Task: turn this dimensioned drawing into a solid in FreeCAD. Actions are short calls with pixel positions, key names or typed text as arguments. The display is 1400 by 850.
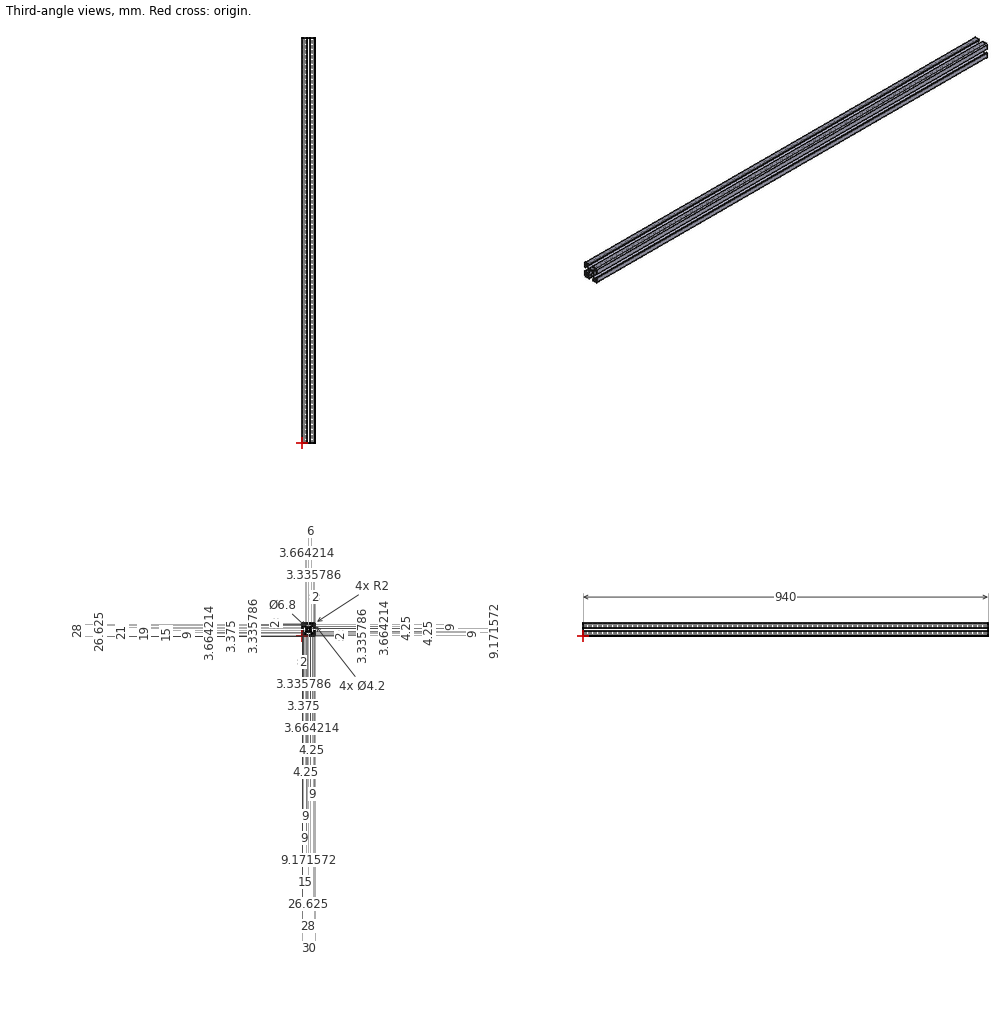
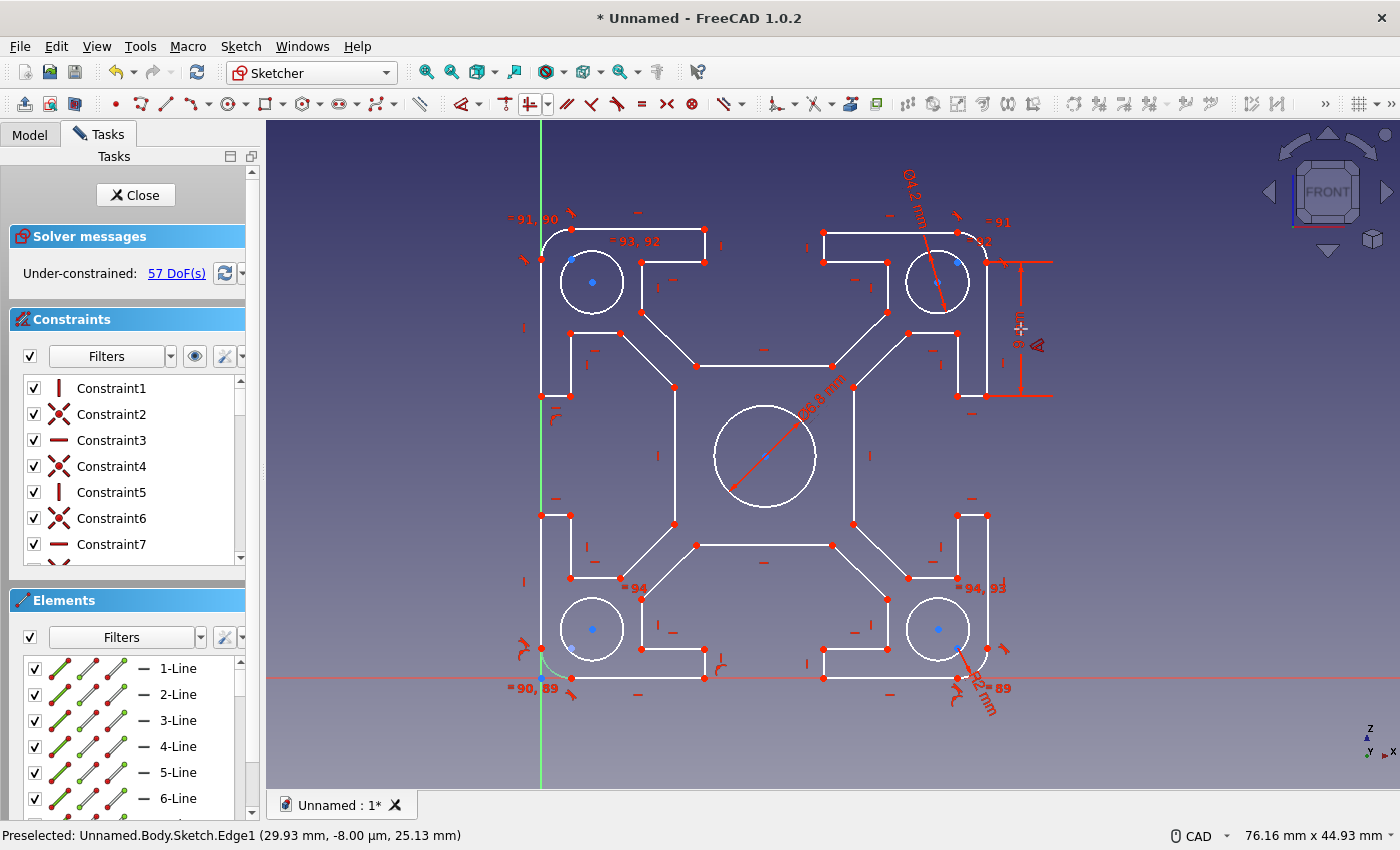
scroll(975, 396, up, 2)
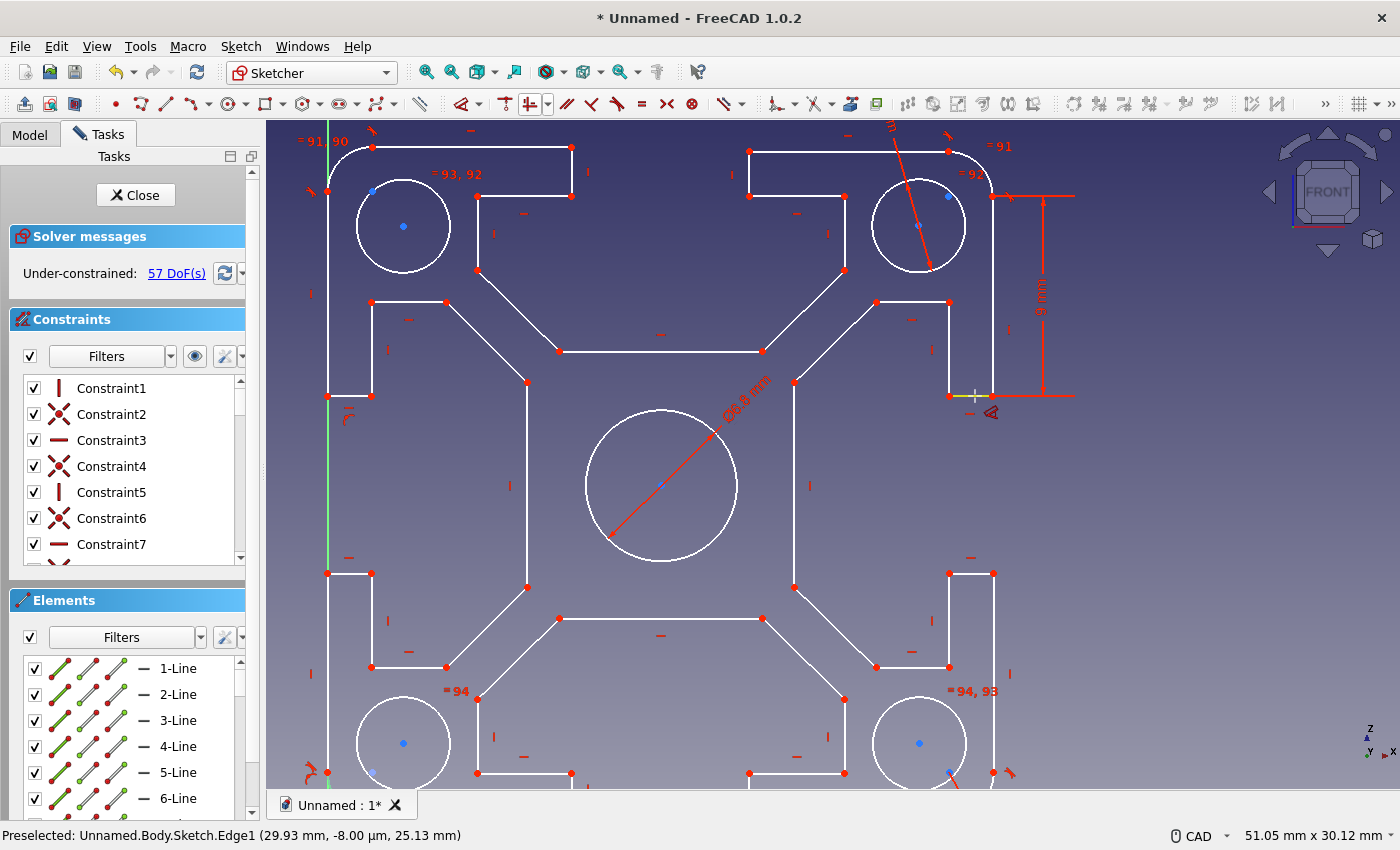
click(975, 396)
click(971, 362)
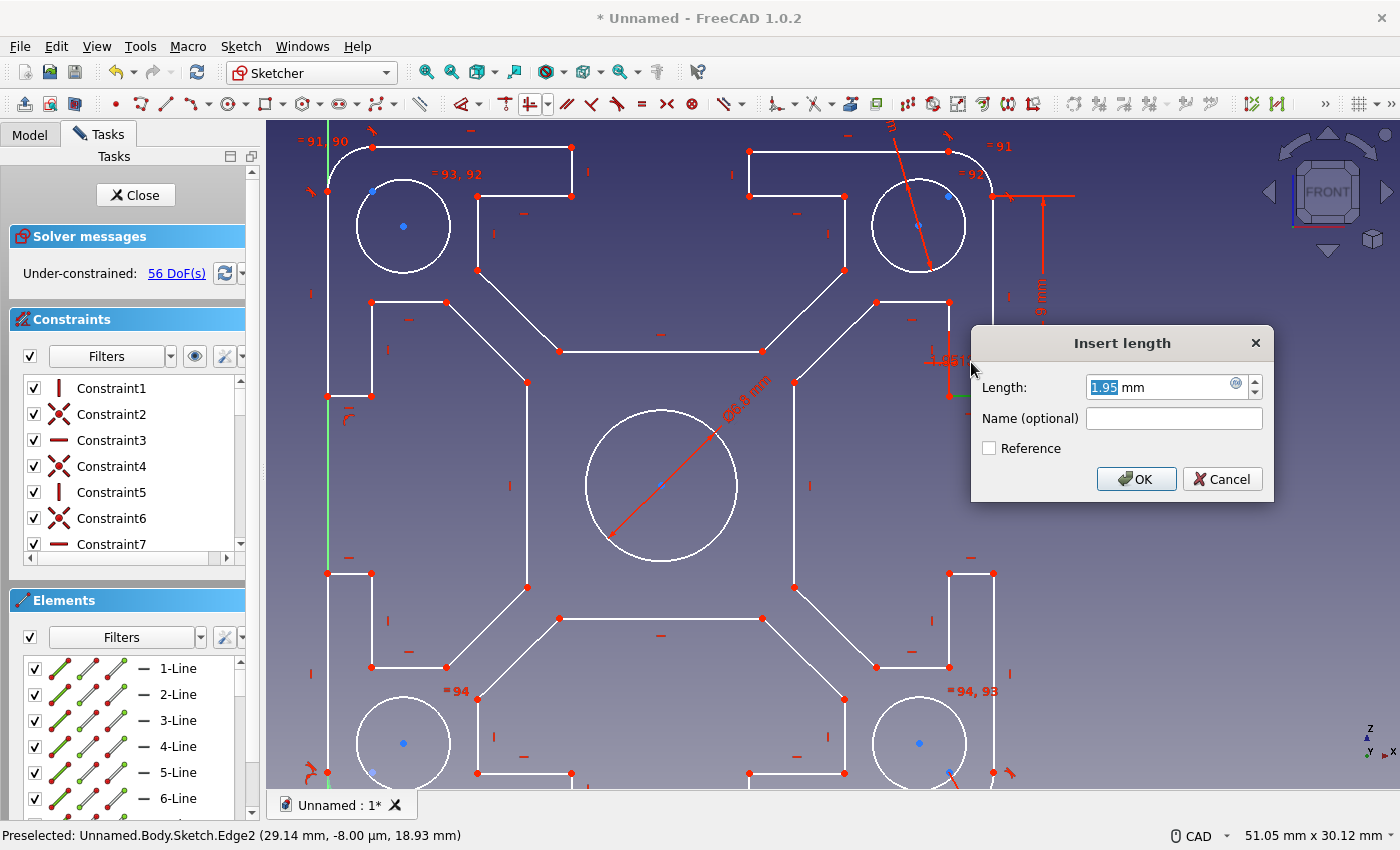
text(2)
key(Return)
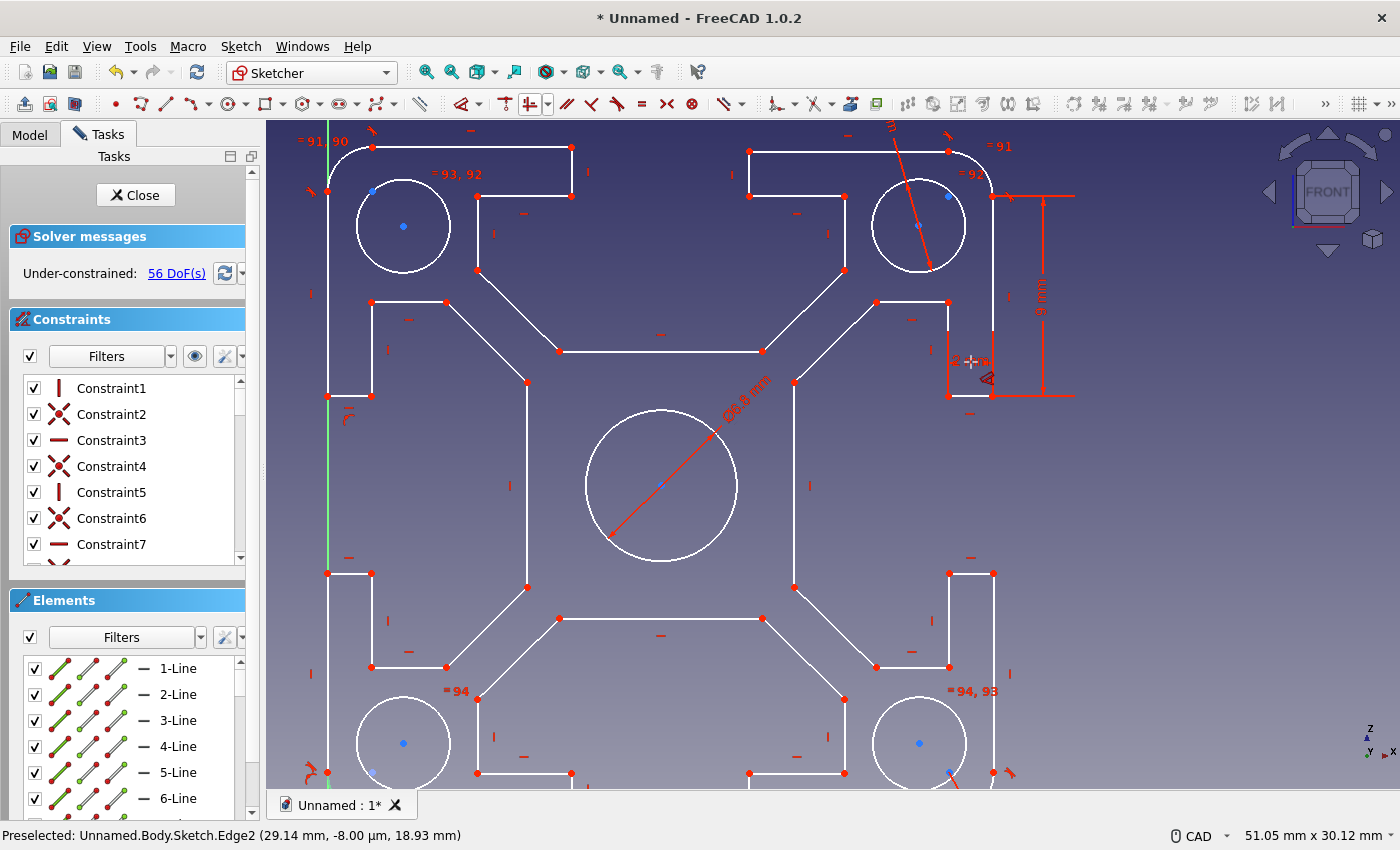
click(963, 574)
click(971, 608)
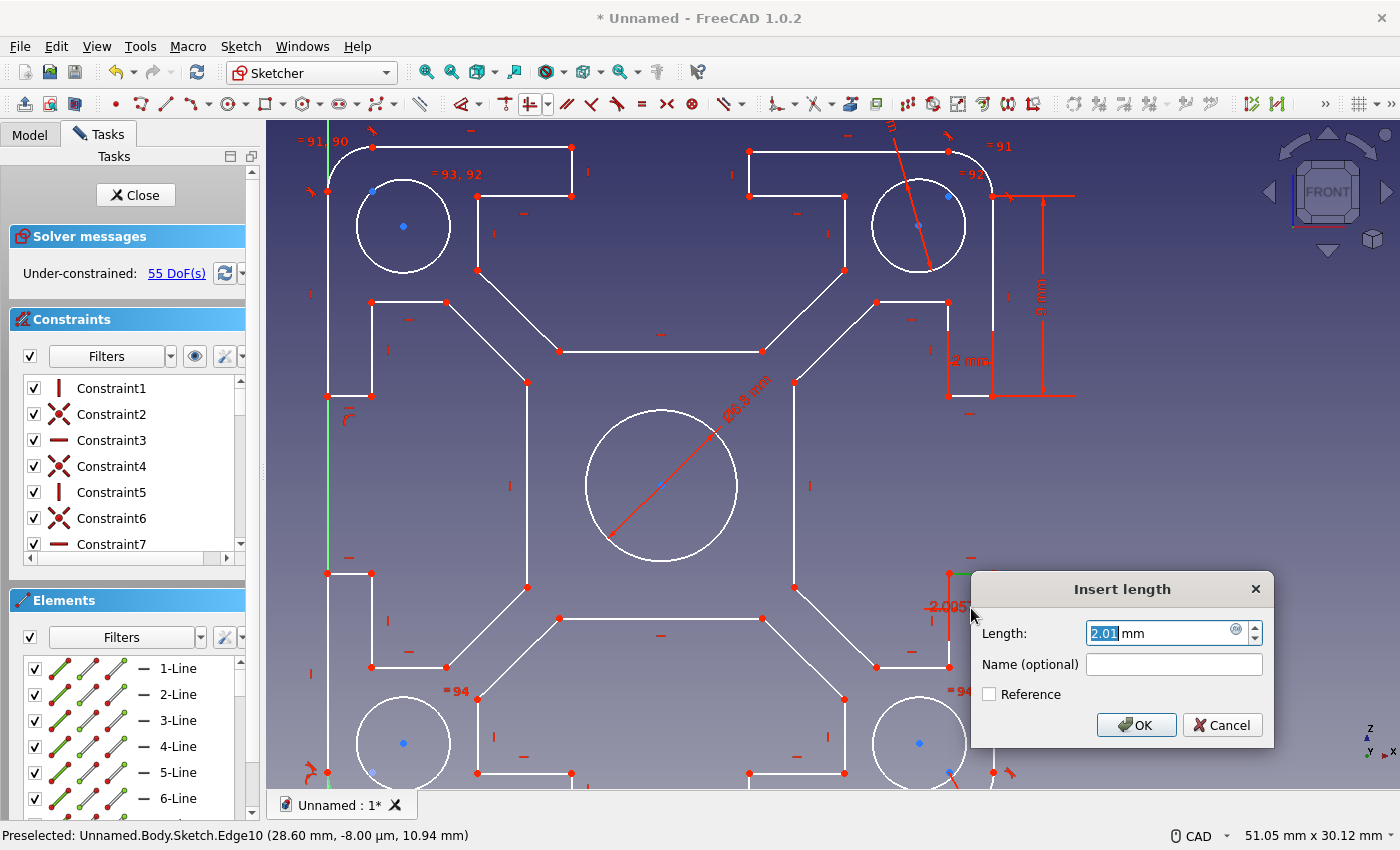
text(2)
key(Return)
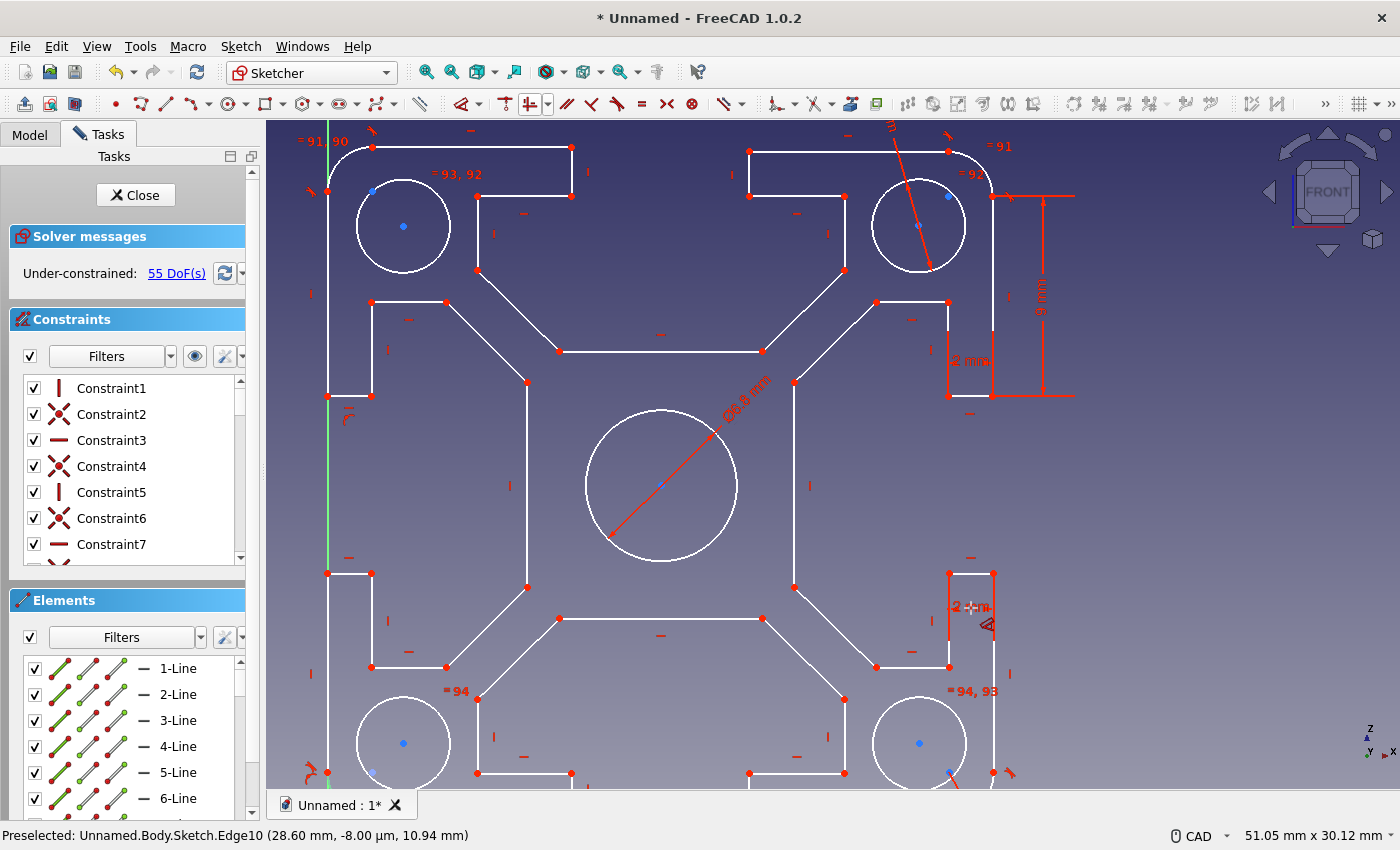
click(994, 633)
click(1028, 667)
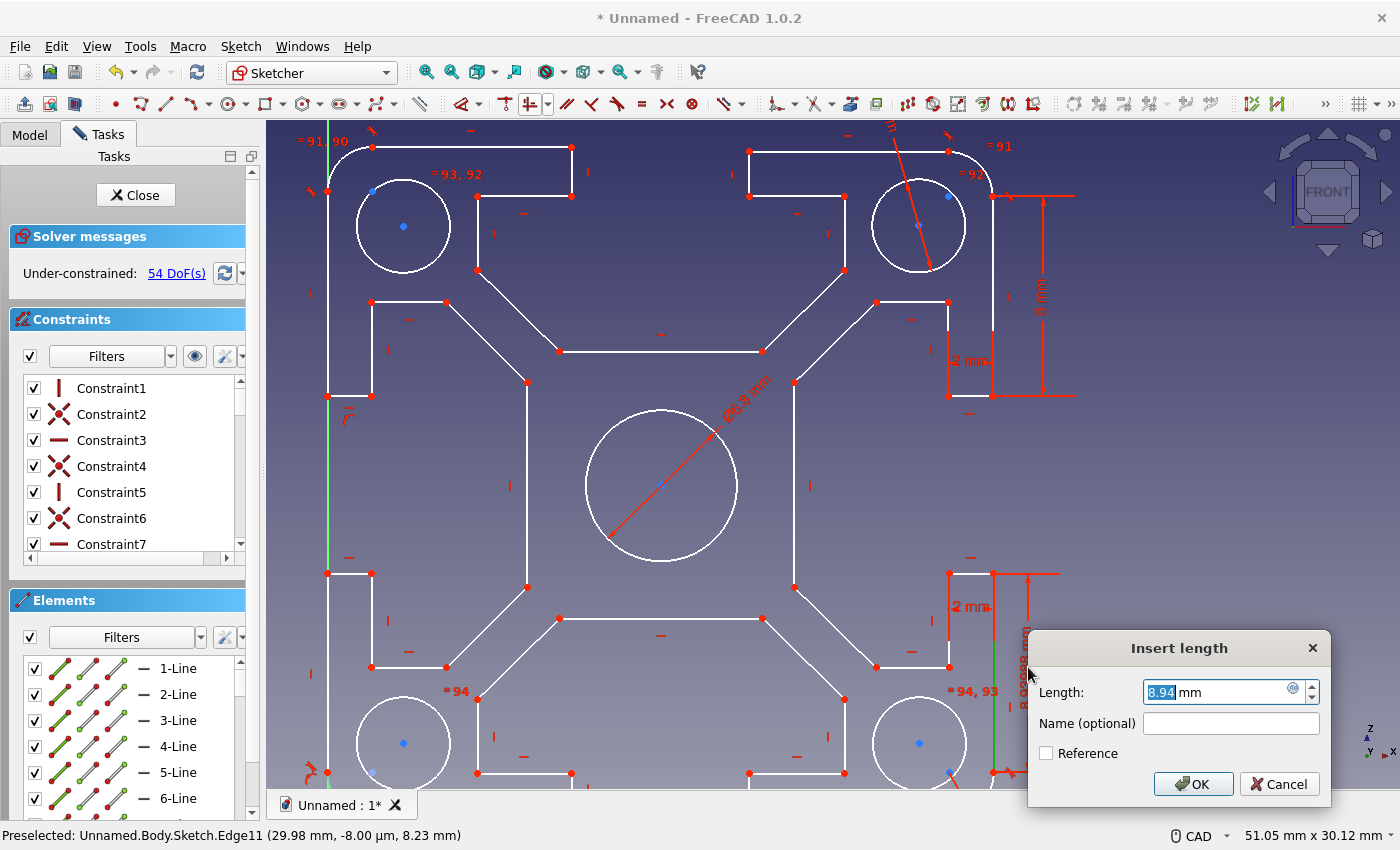
text(9)
key(Return)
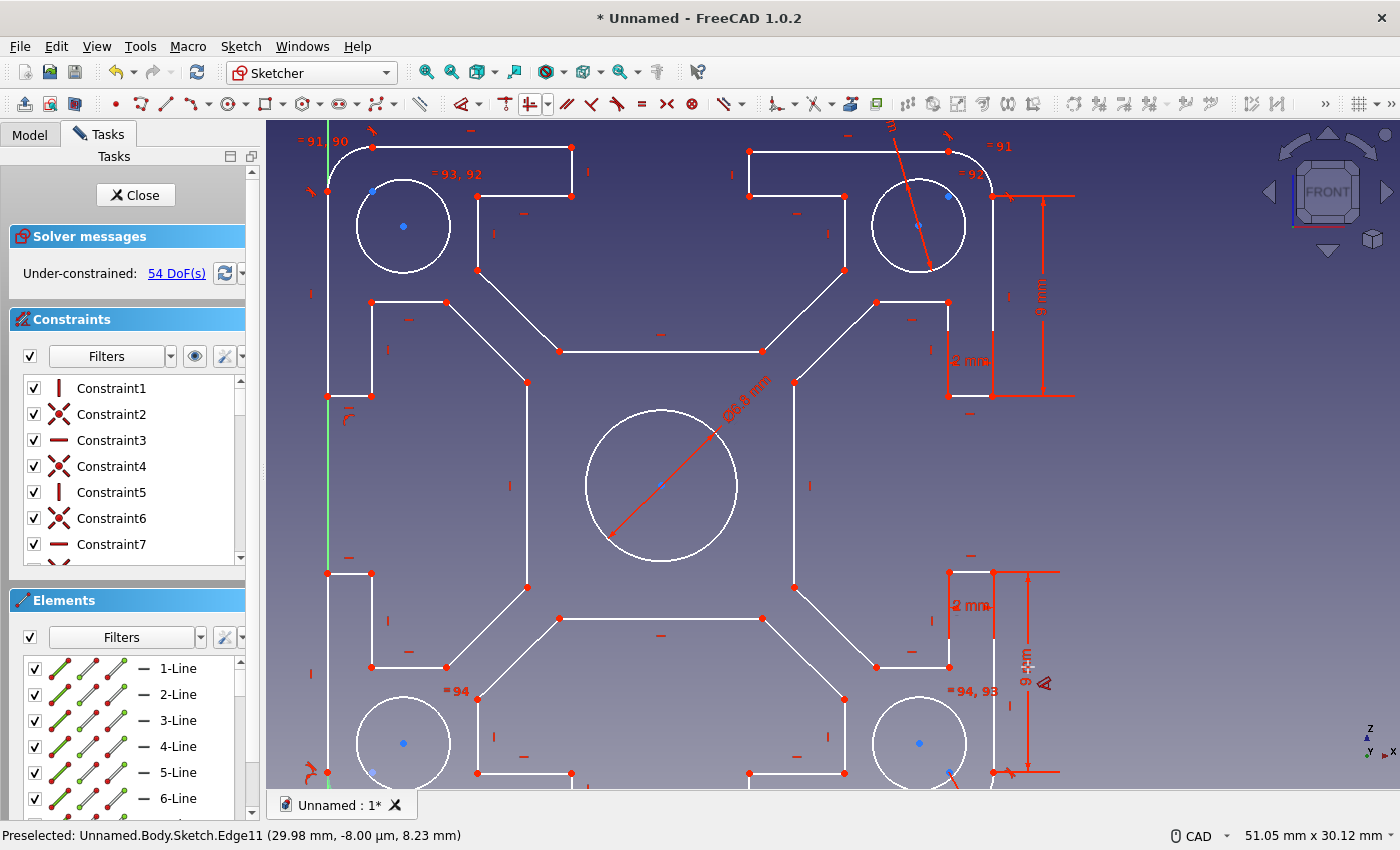
scroll(975, 395, down, 2)